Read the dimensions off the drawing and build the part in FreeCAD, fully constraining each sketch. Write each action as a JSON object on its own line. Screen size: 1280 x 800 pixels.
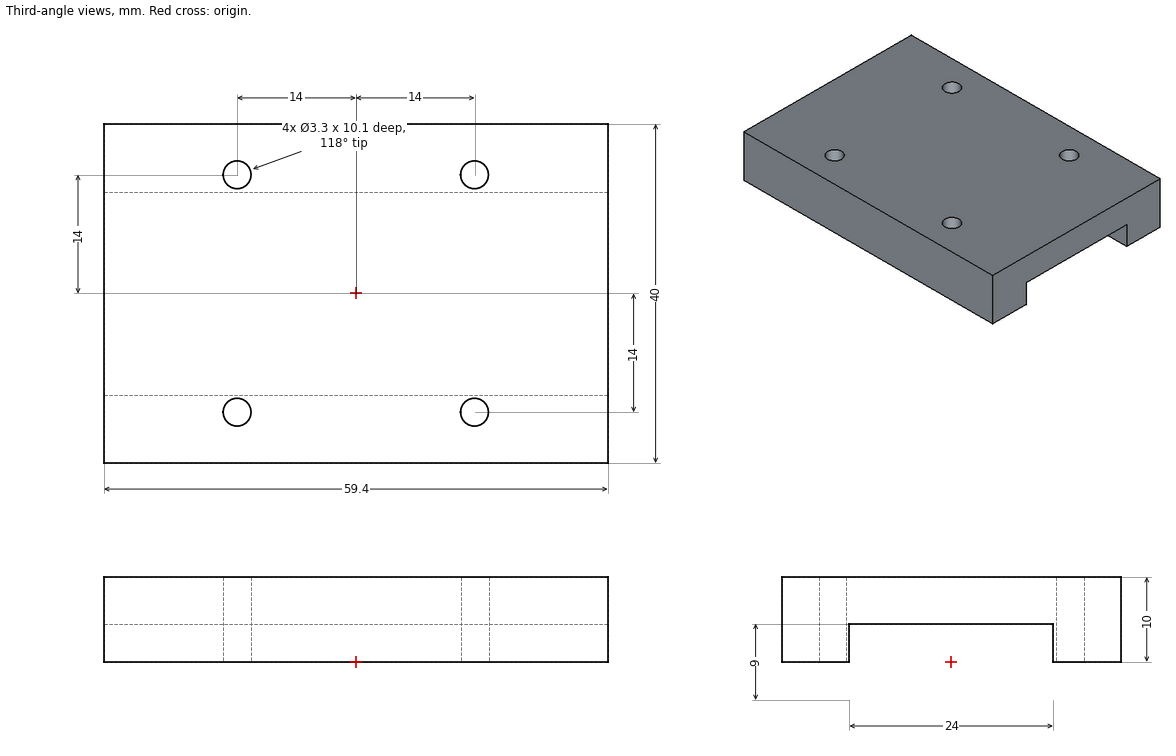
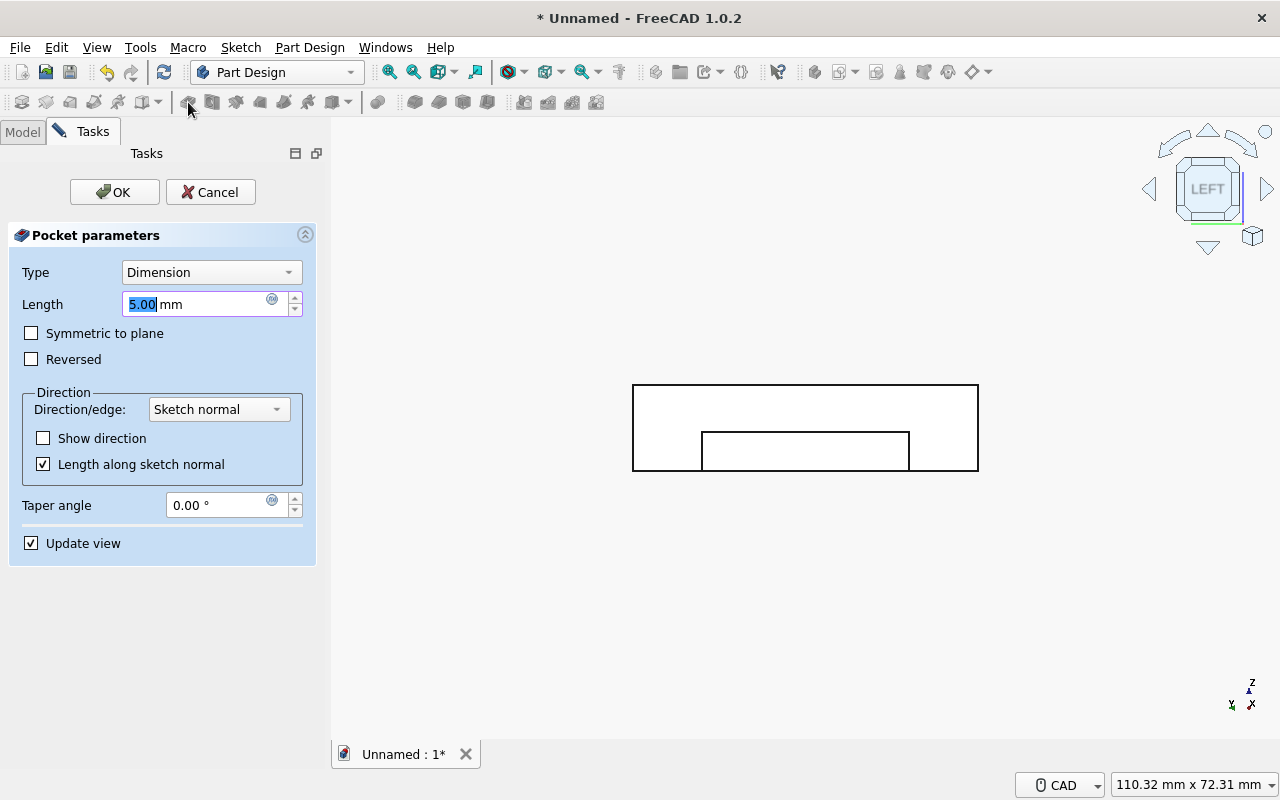
{"action": "left_click", "coordinate": [212, 272]}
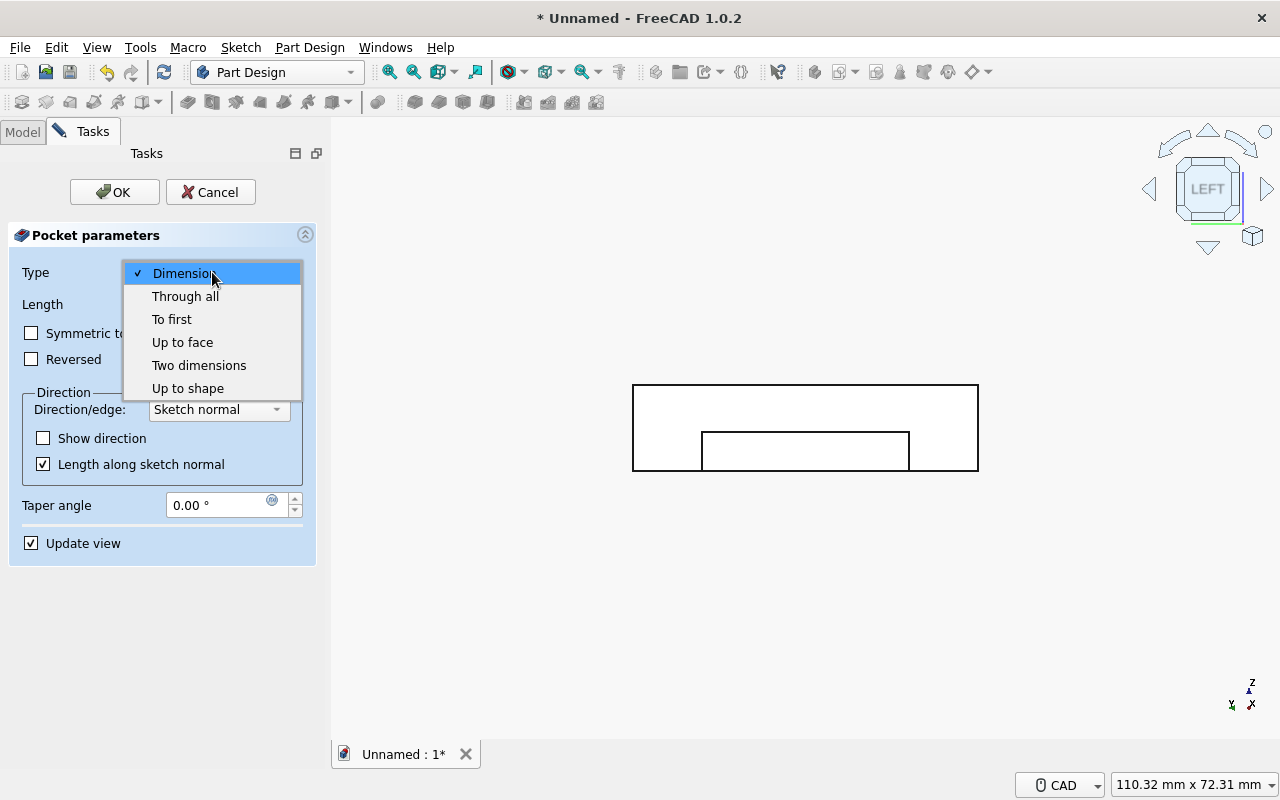
{"action": "left_click", "coordinate": [212, 296]}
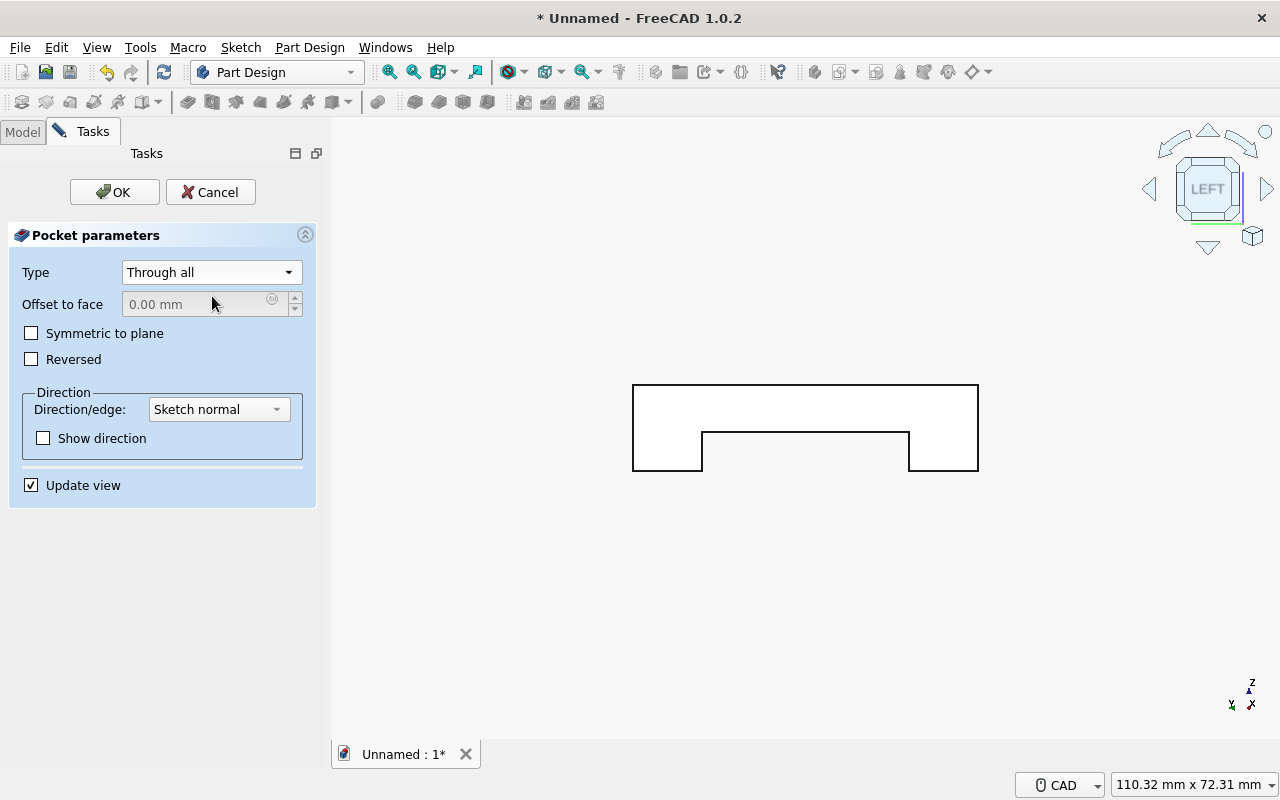
{"action": "left_click", "coordinate": [115, 192]}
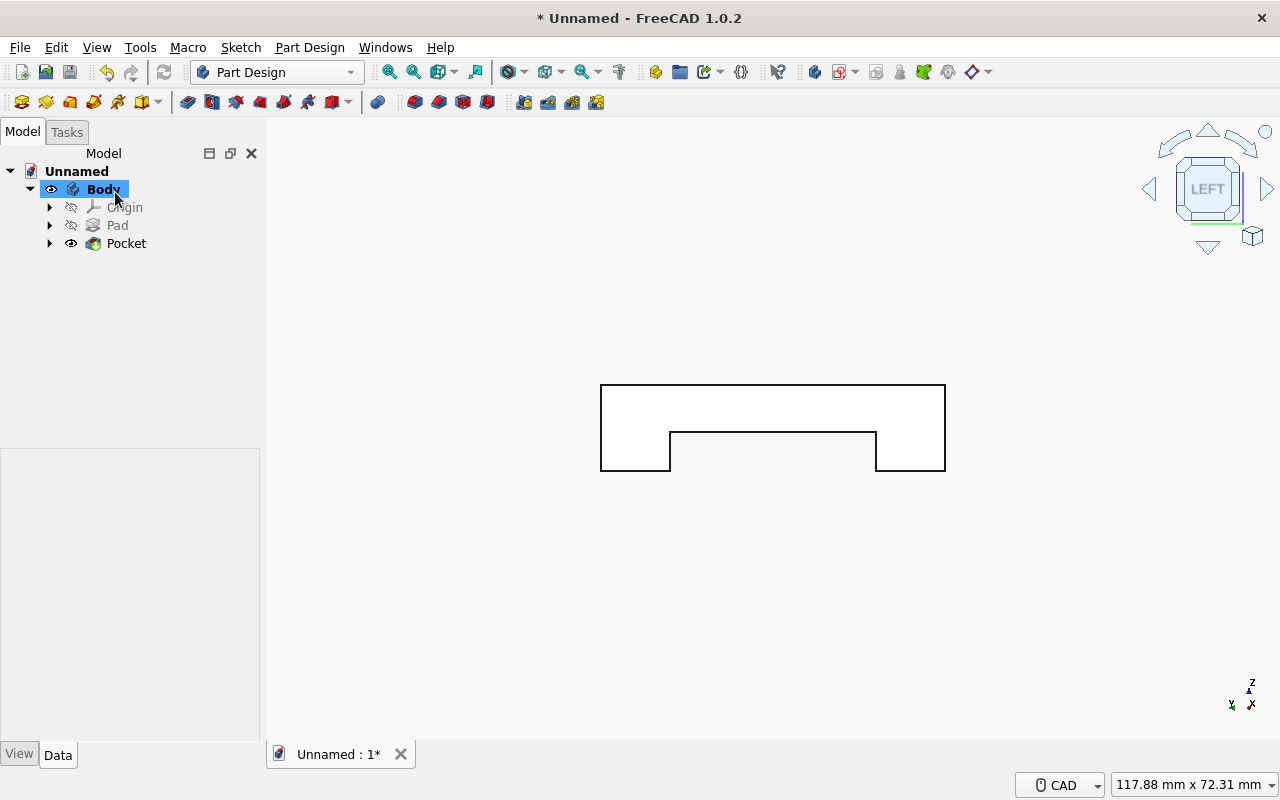
{"action": "key", "text": "v f"}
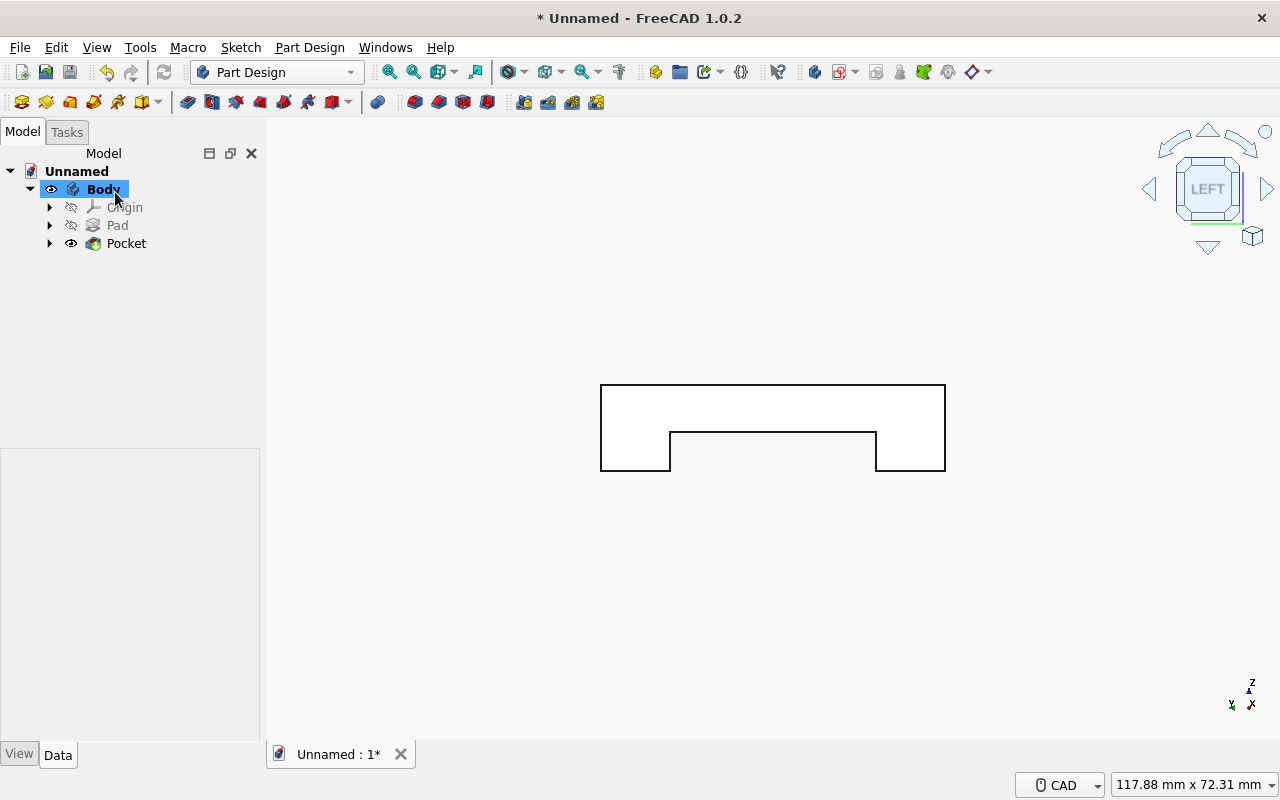
{"action": "key", "text": "0"}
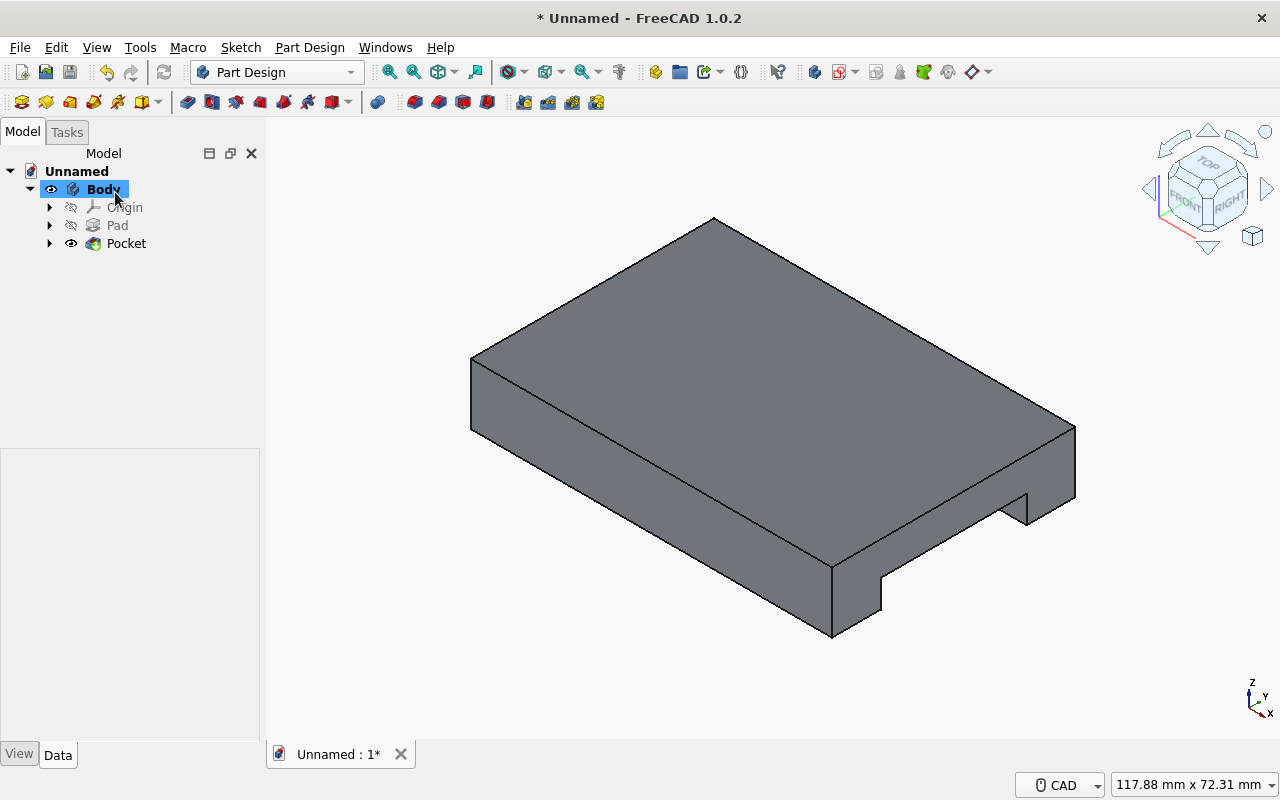
{"action": "left_click", "coordinate": [825, 422]}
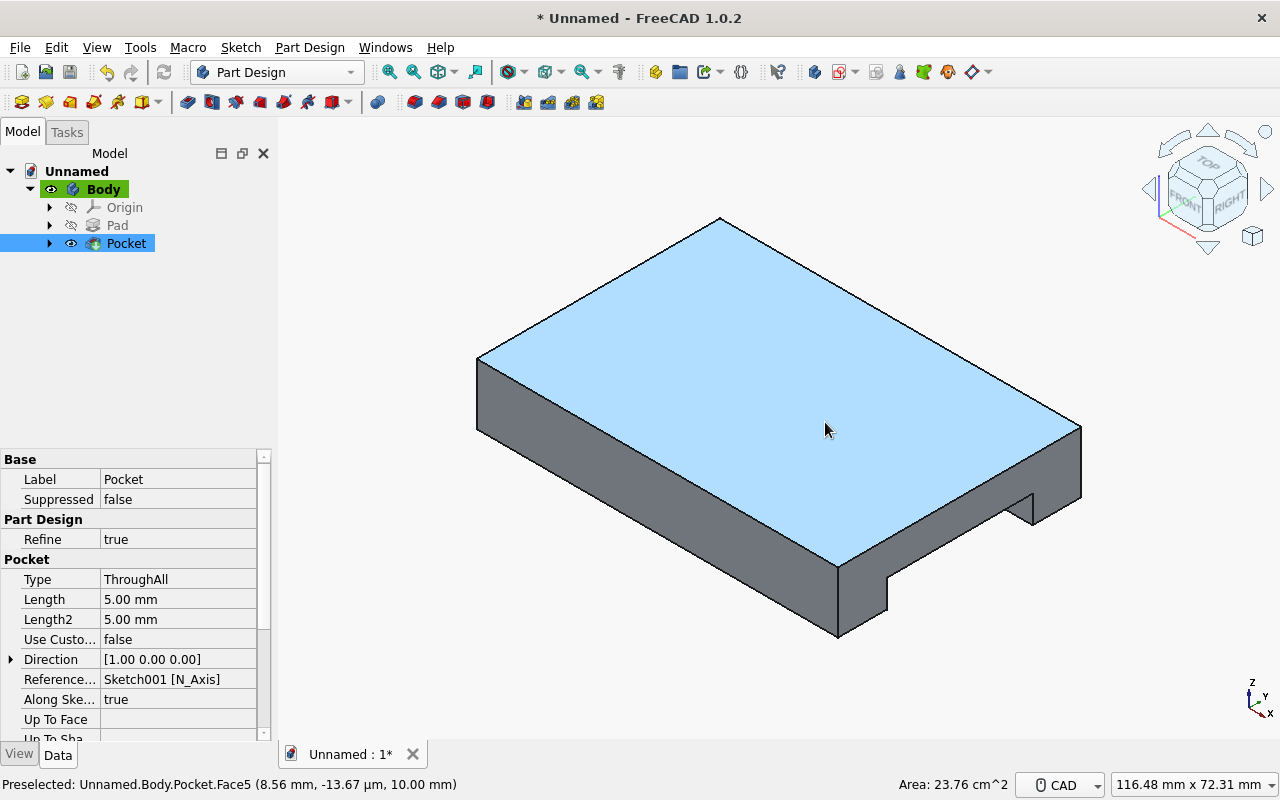
{"action": "left_click", "coordinate": [840, 72]}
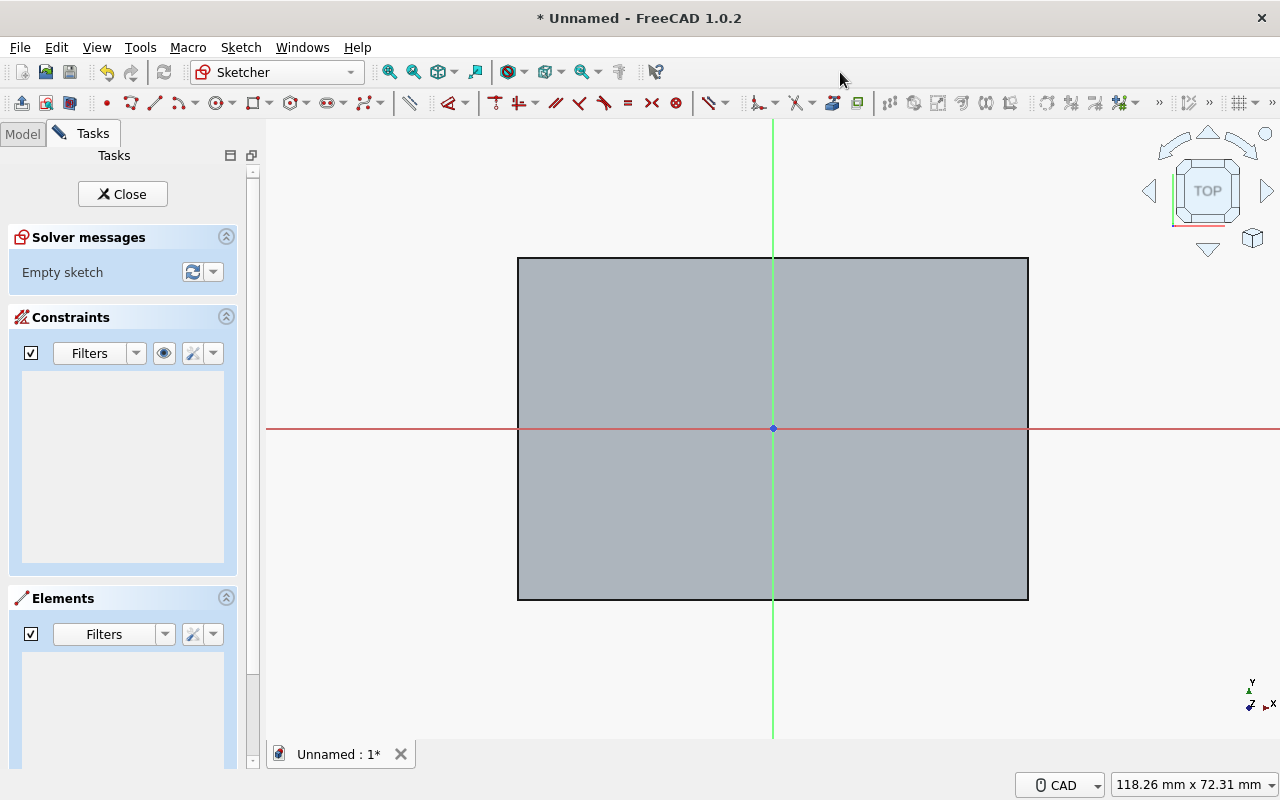
{"action": "scroll", "coordinate": [912, 429], "scroll_direction": "up", "scroll_amount": 2}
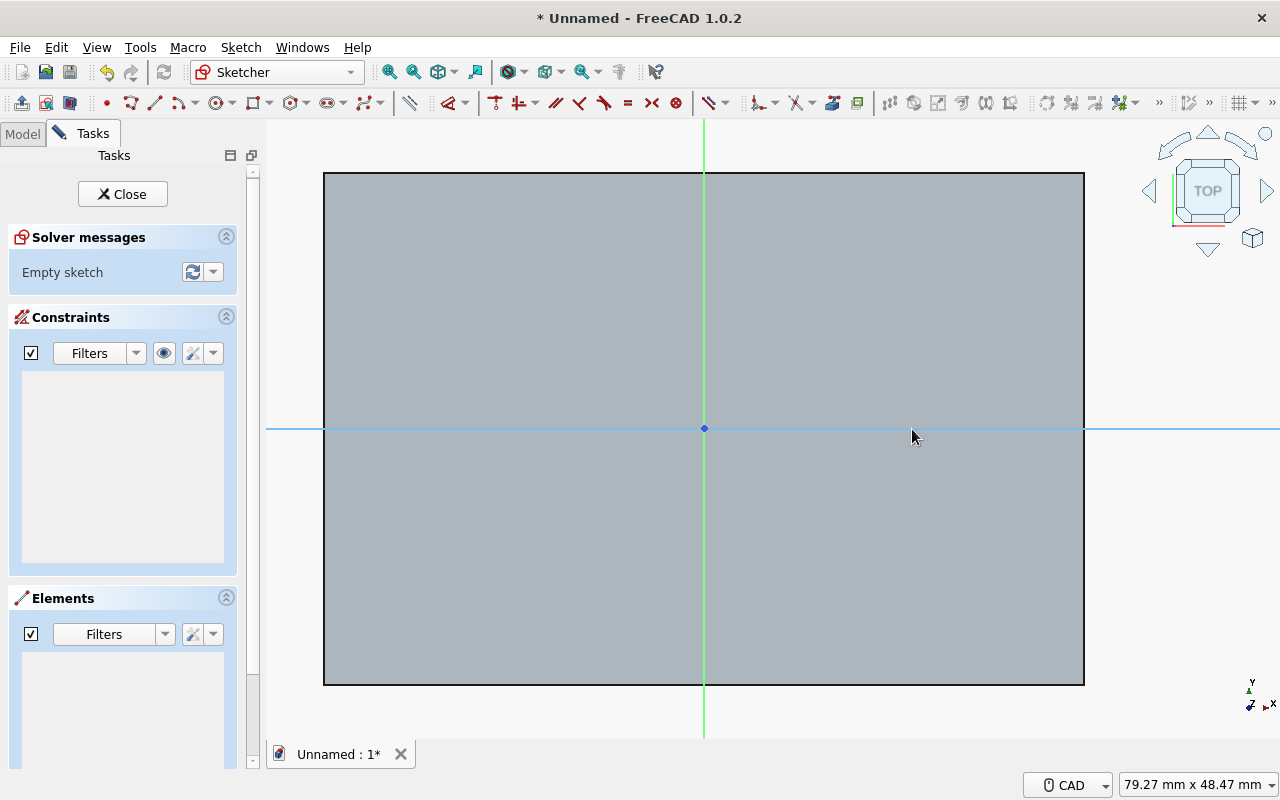
{"action": "left_click", "coordinate": [216, 104]}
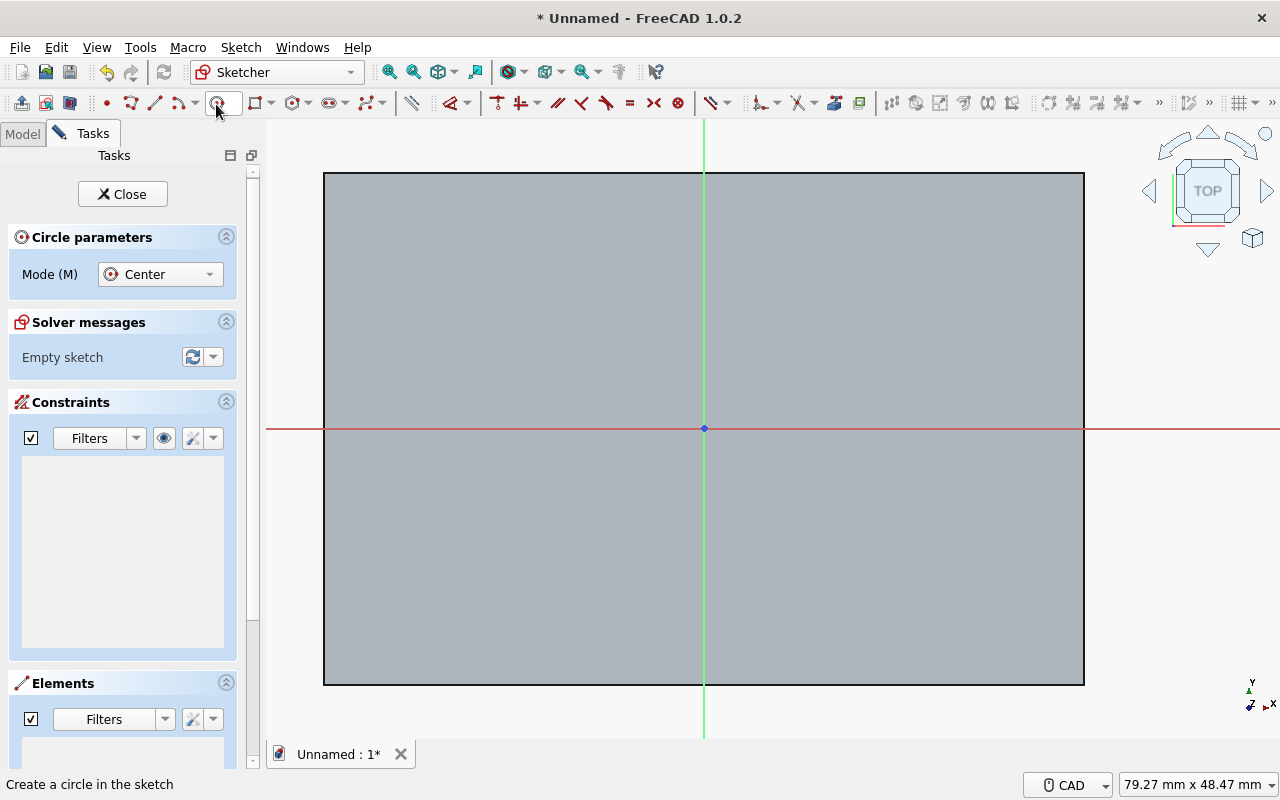
{"action": "left_click", "coordinate": [525, 250]}
{"action": "left_click", "coordinate": [540, 235]}